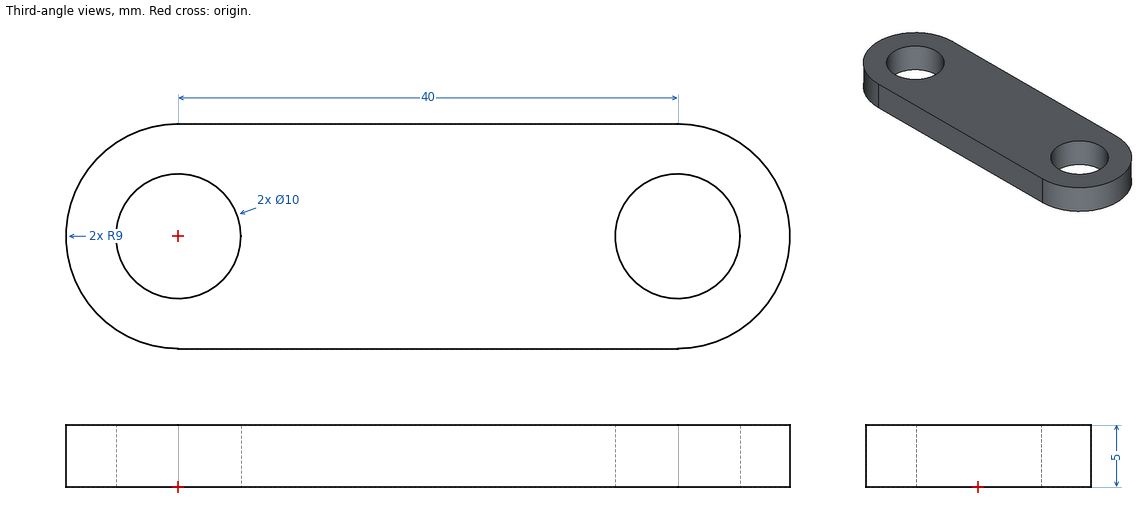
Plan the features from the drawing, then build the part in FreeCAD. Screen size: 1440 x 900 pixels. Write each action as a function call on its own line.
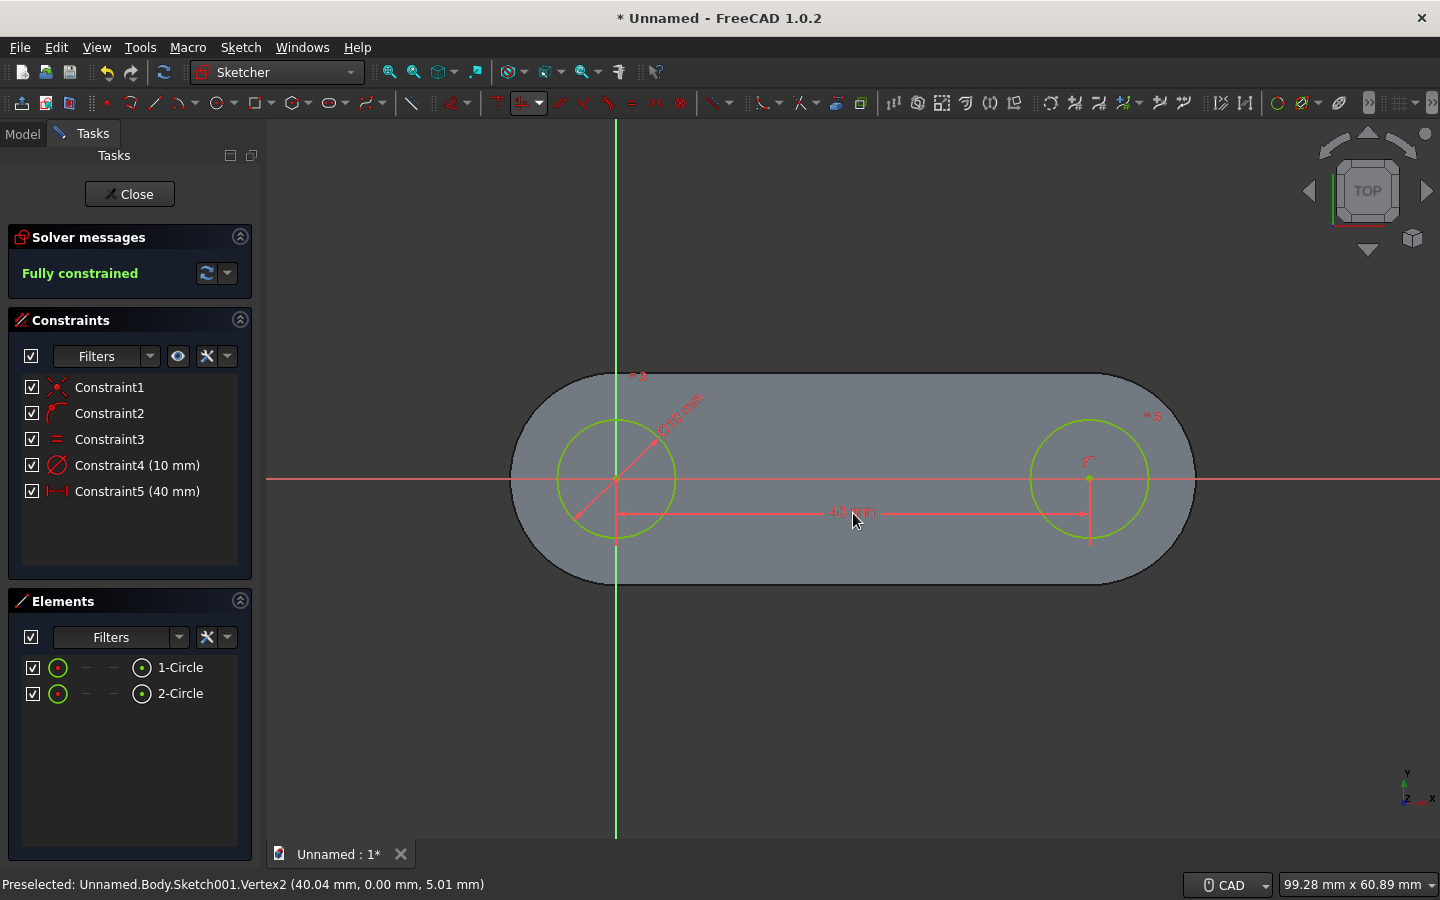
click(130, 194)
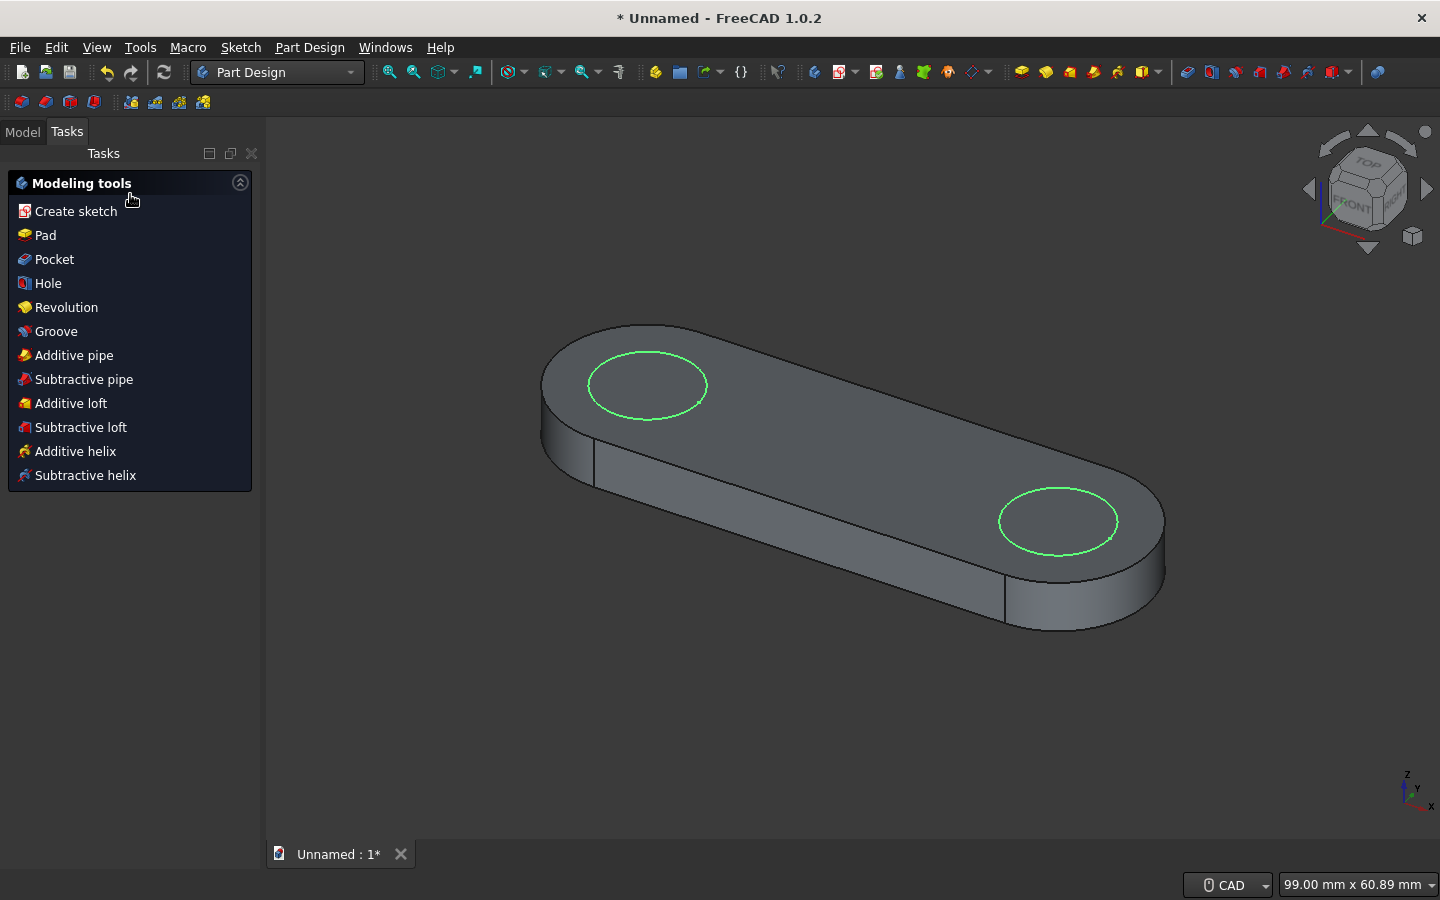
click(1188, 72)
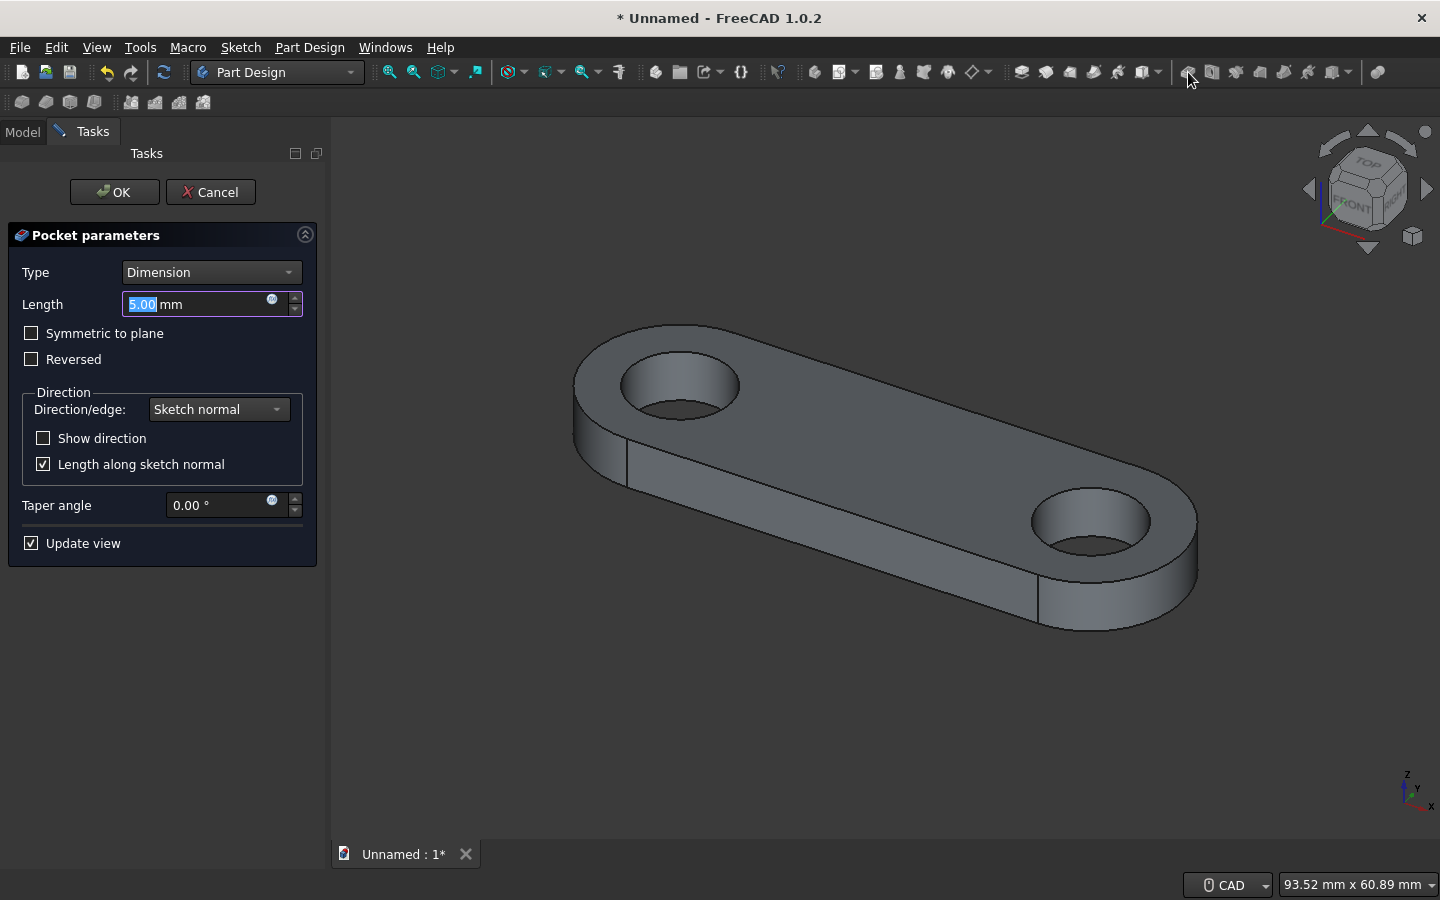
click(212, 272)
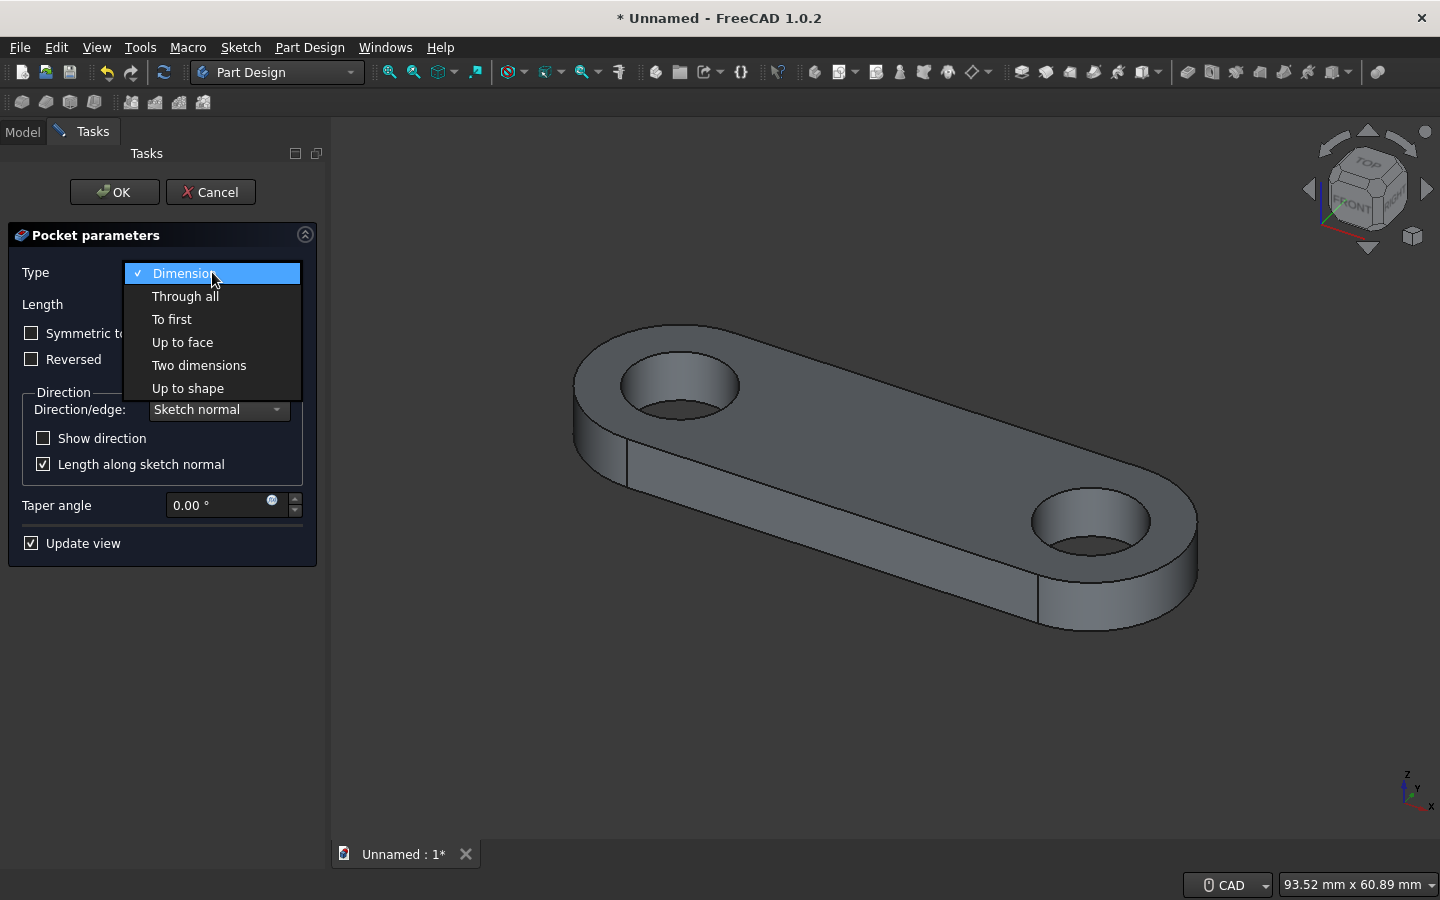
click(212, 296)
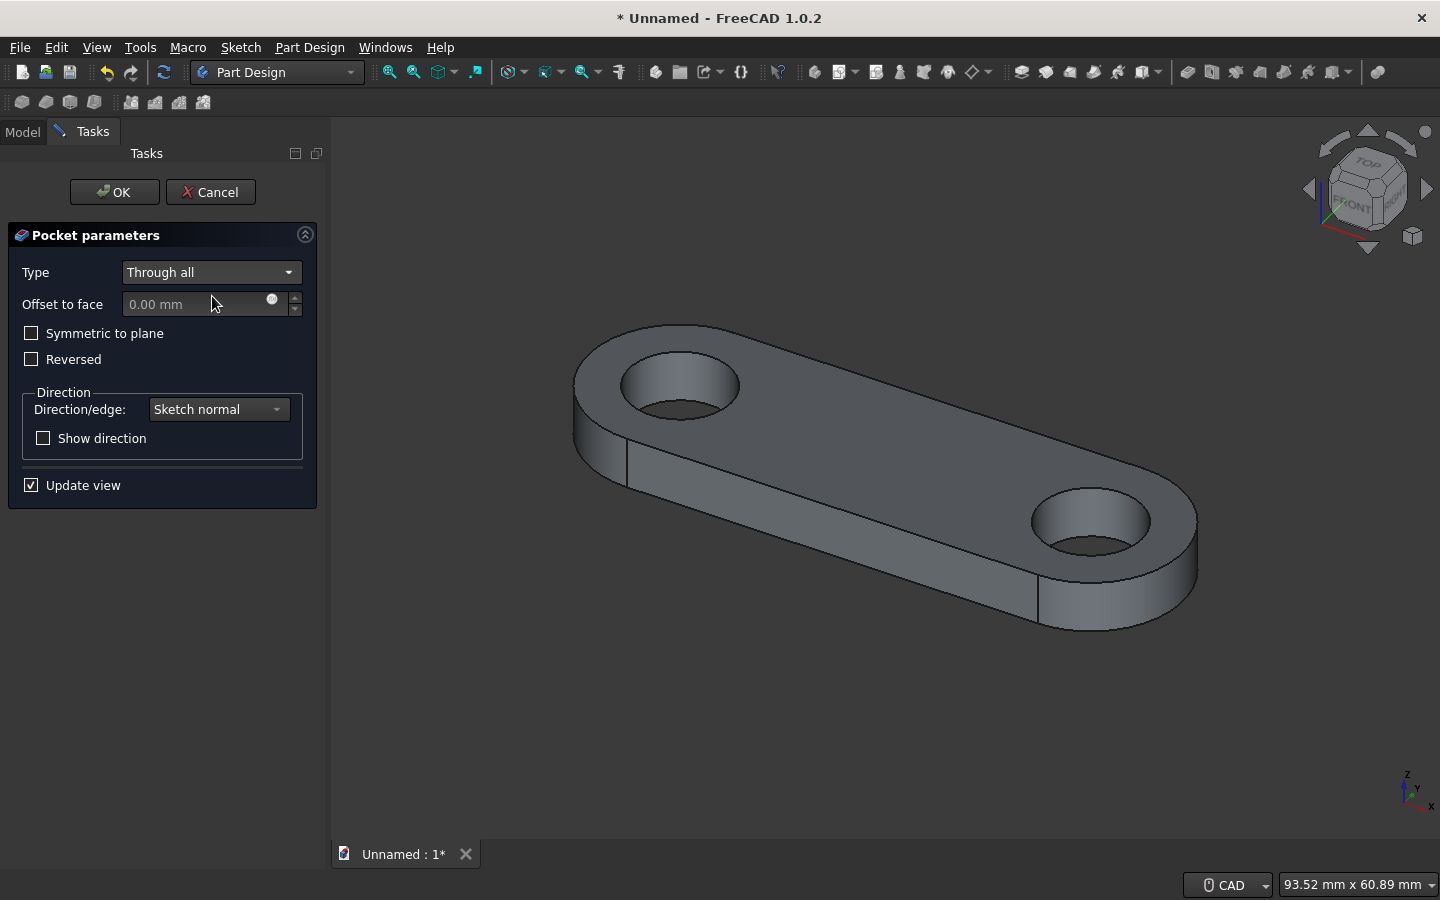
click(115, 192)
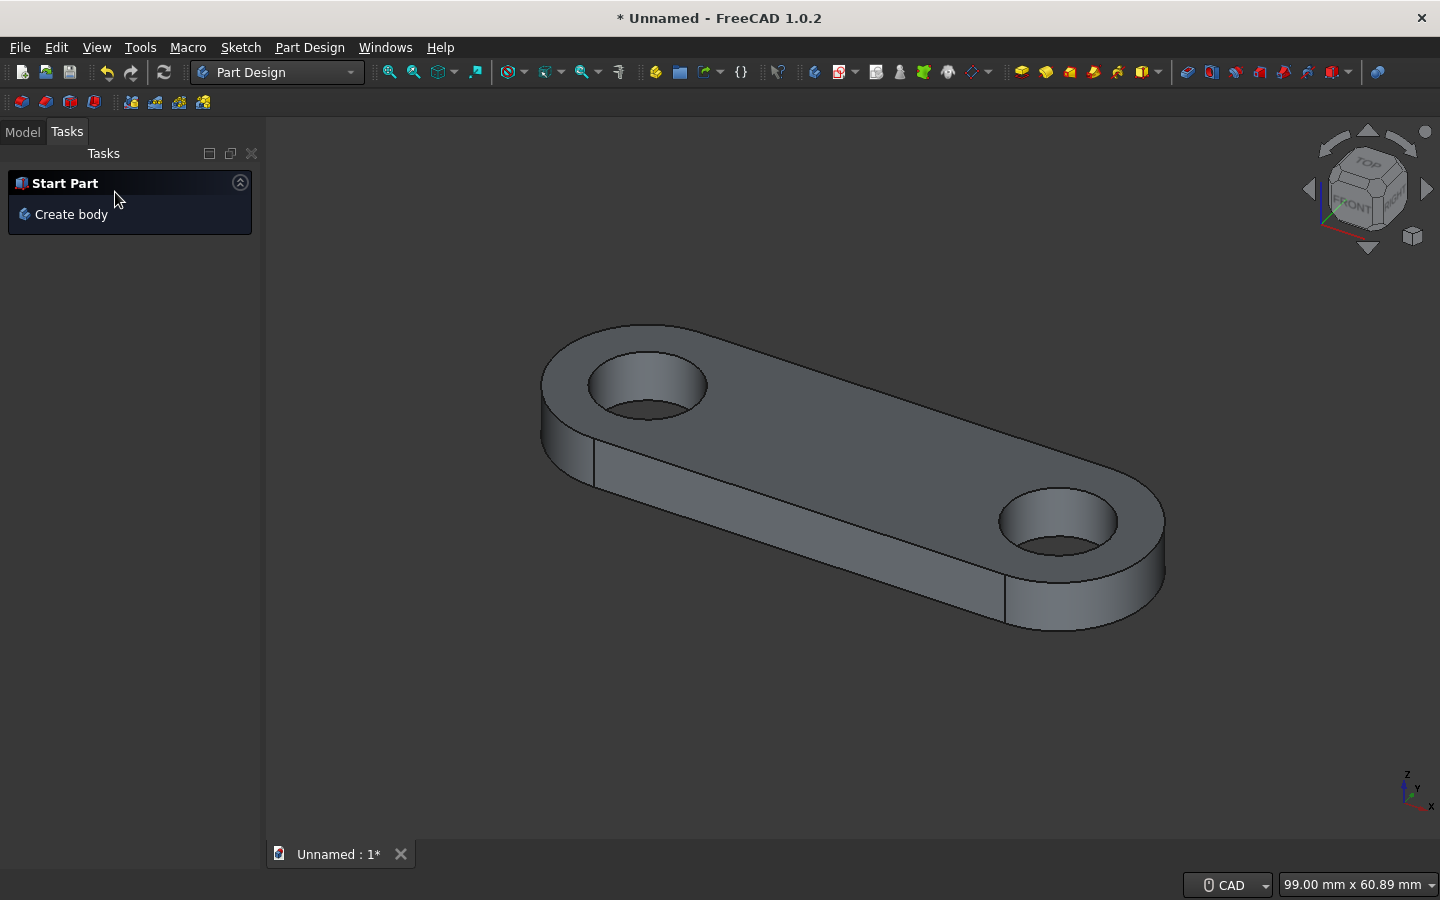
key(0)